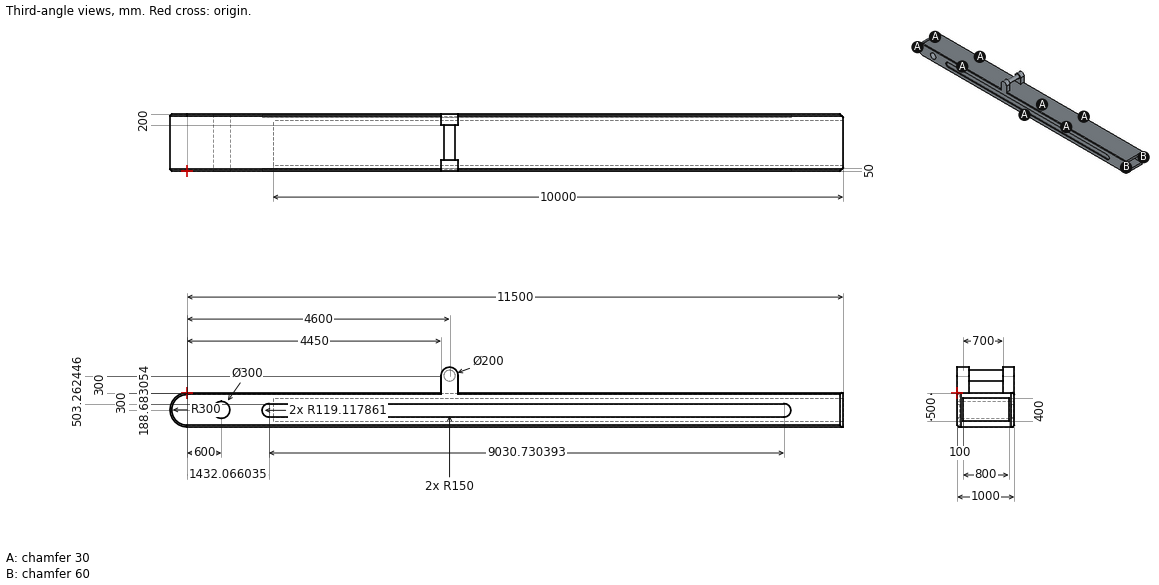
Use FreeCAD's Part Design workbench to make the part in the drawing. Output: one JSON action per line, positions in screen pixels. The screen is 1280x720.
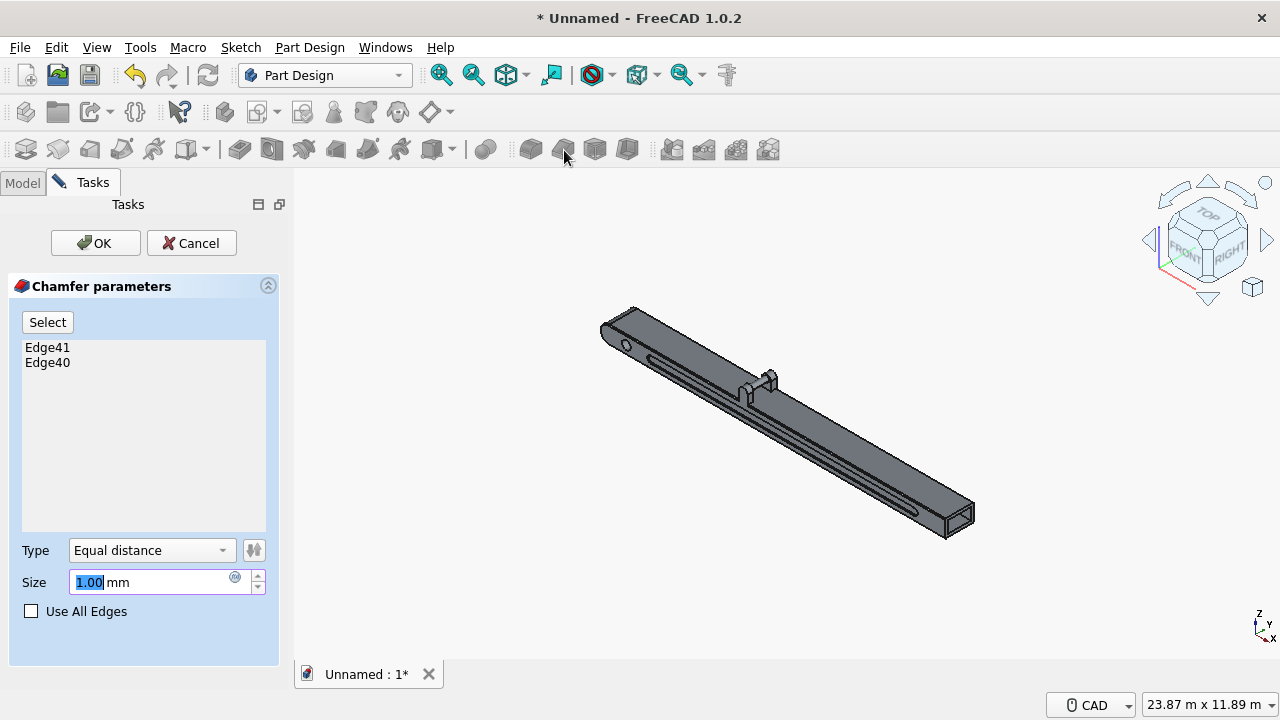
{"action": "type", "text": "60"}
{"action": "key", "text": "Tab"}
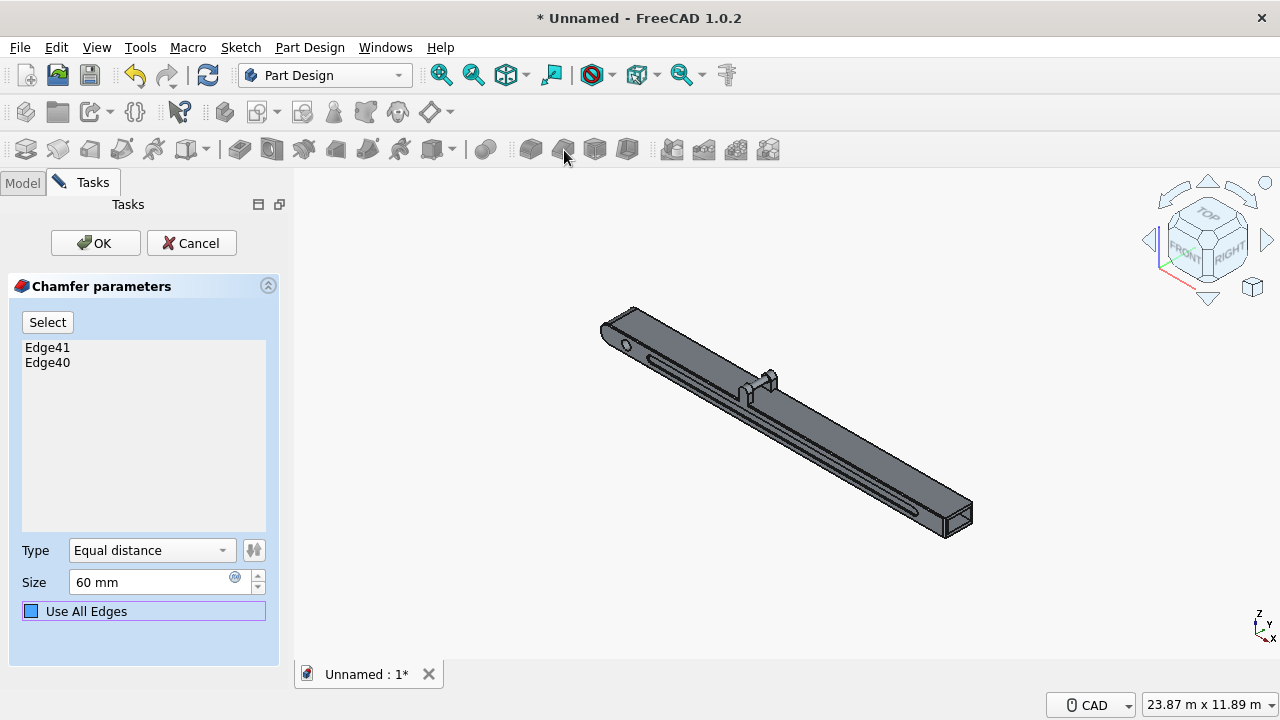
{"action": "left_click", "coordinate": [96, 243]}